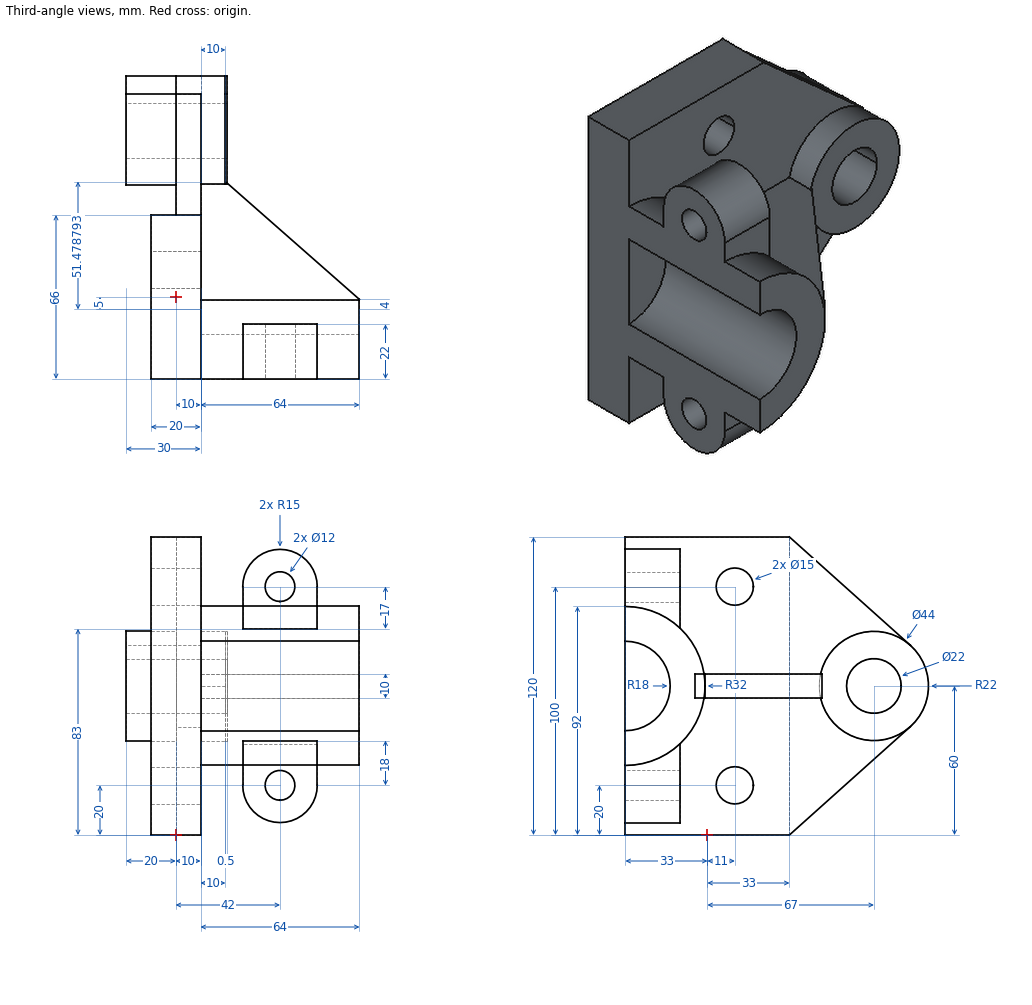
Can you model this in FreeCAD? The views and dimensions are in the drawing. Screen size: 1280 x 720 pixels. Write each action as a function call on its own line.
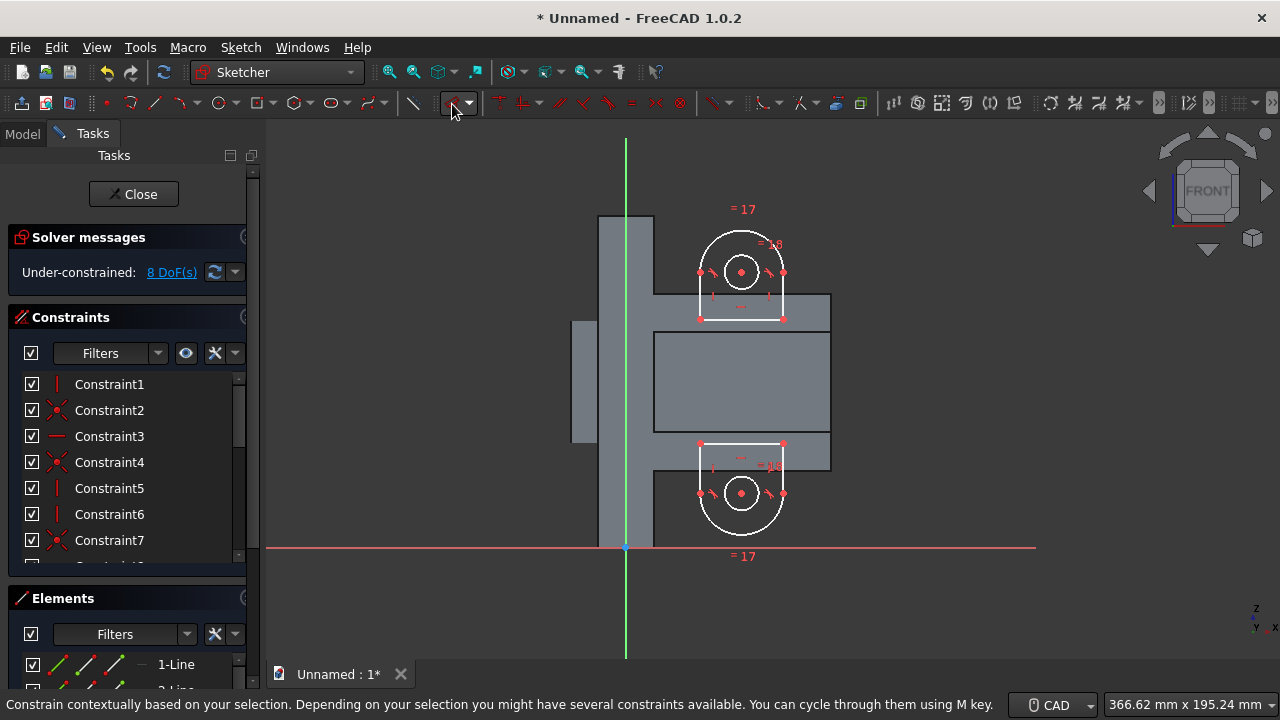
click(766, 239)
click(785, 213)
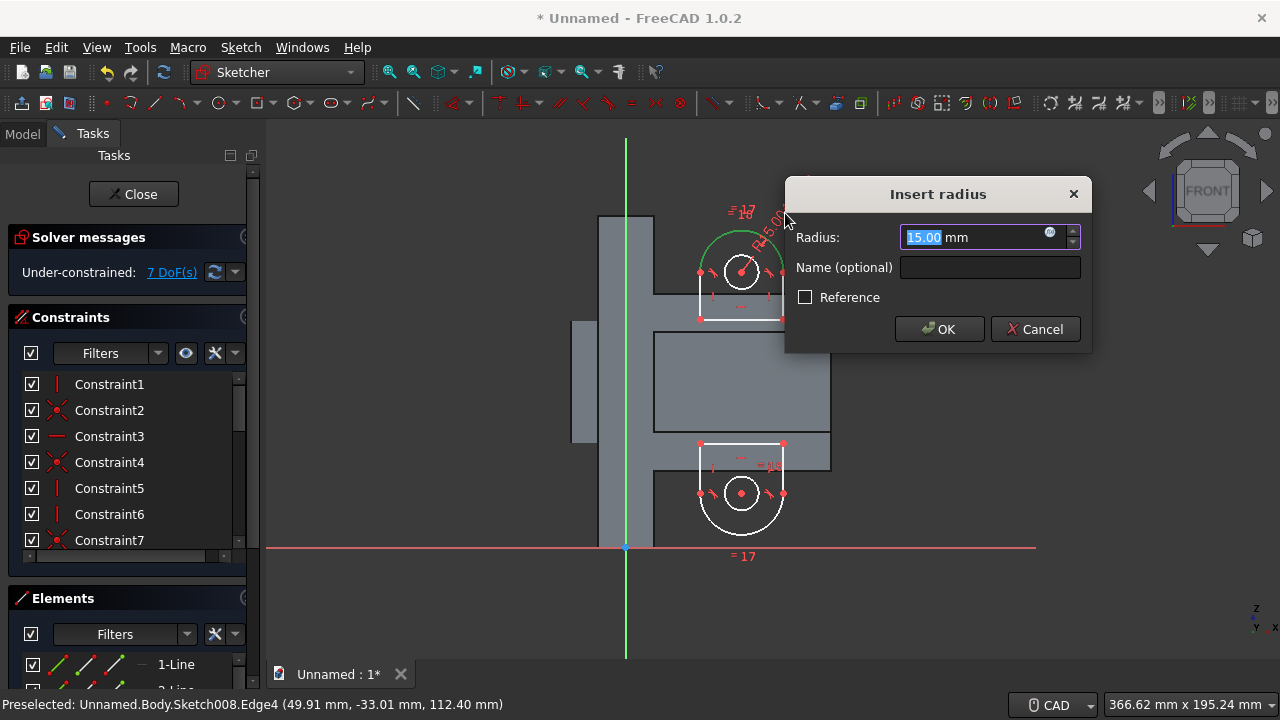
text(15)
key(Return)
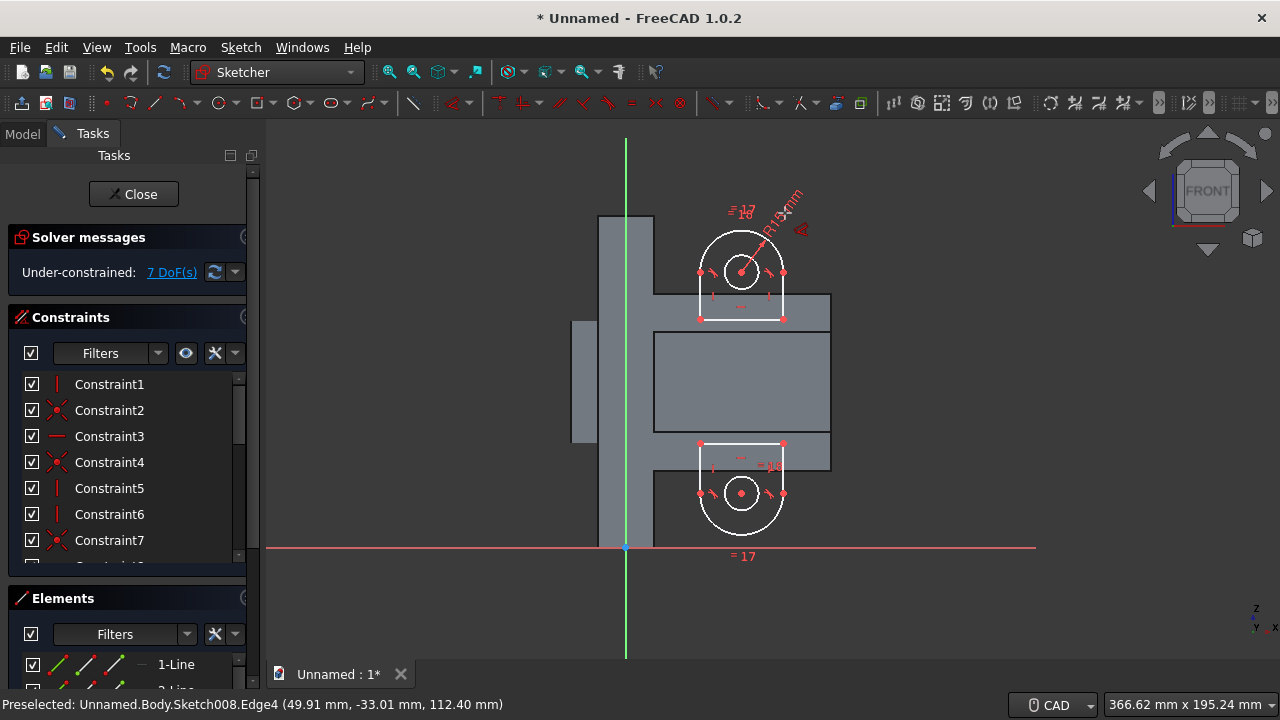
click(754, 260)
click(811, 252)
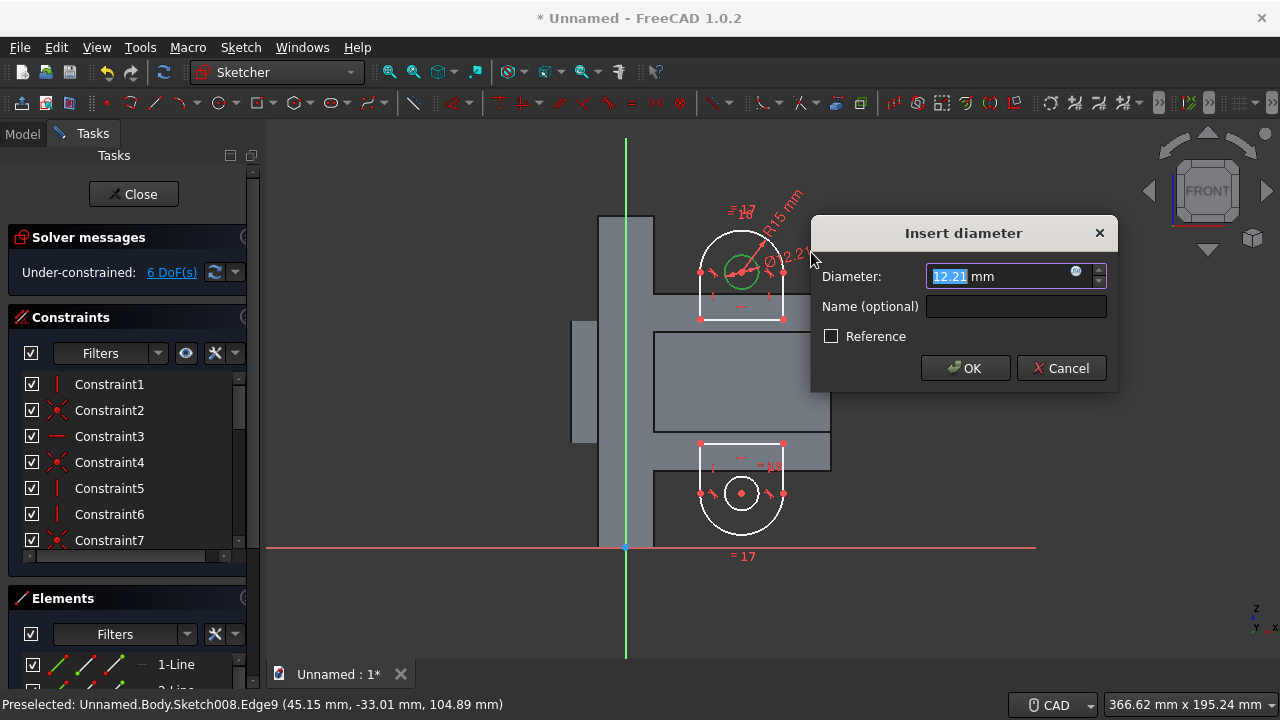
text(12)
key(Return)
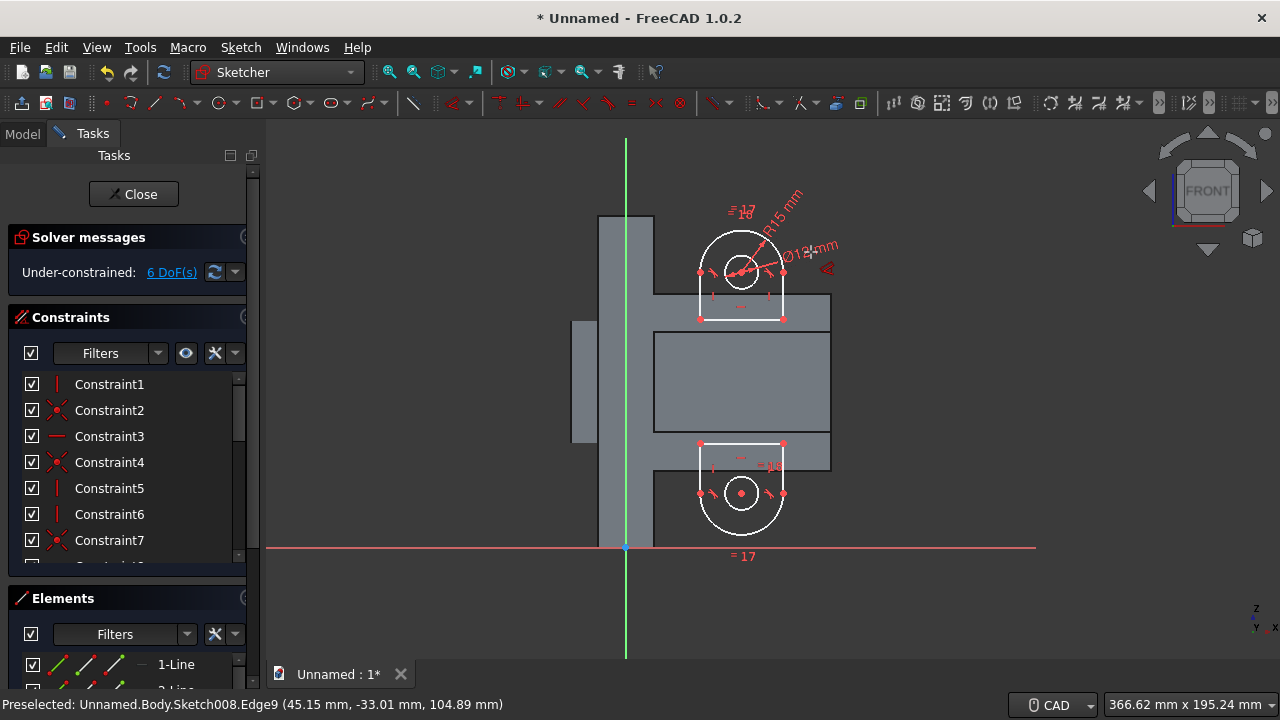
click(700, 286)
click(666, 296)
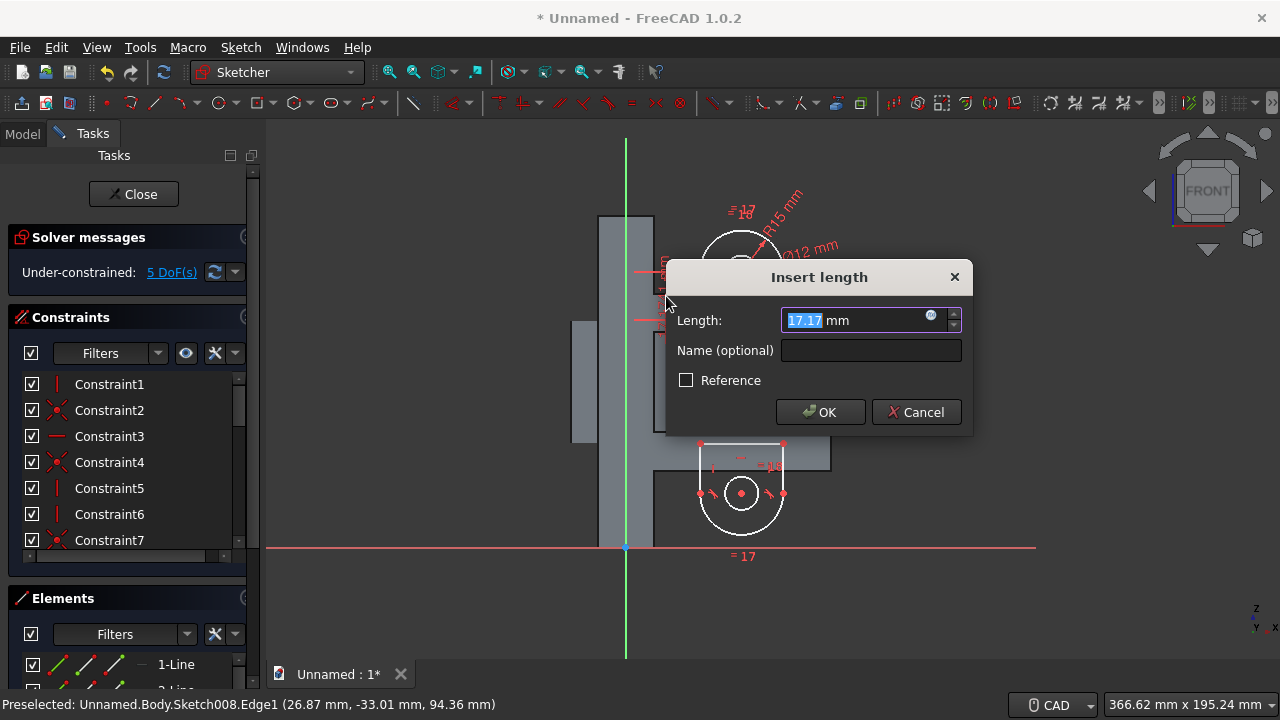
text(17)
key(Return)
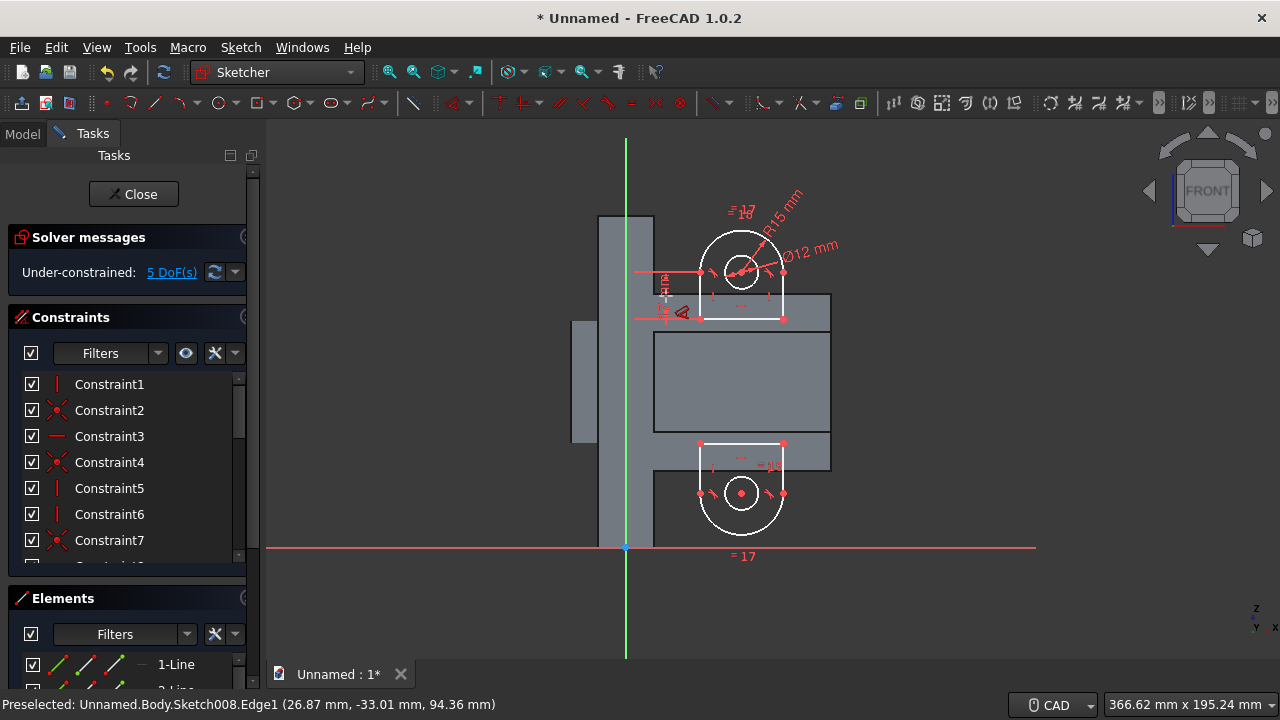
click(783, 478)
click(817, 469)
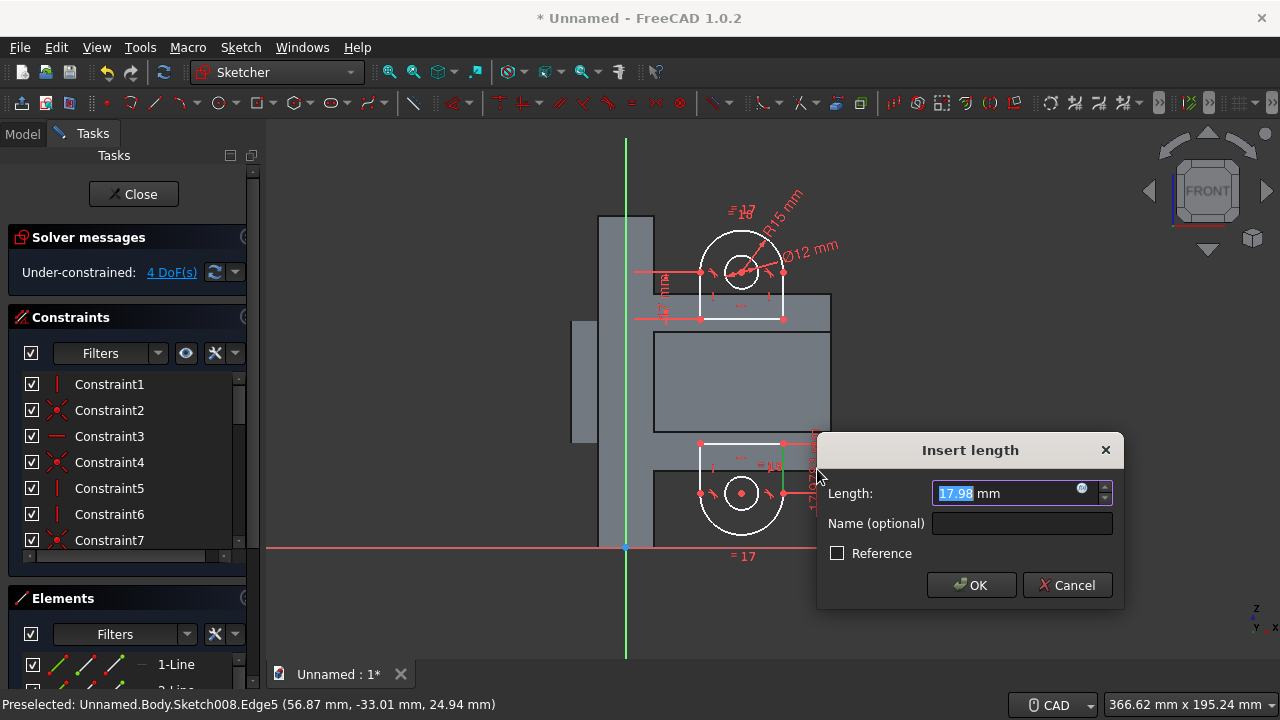
text(18)
key(Return)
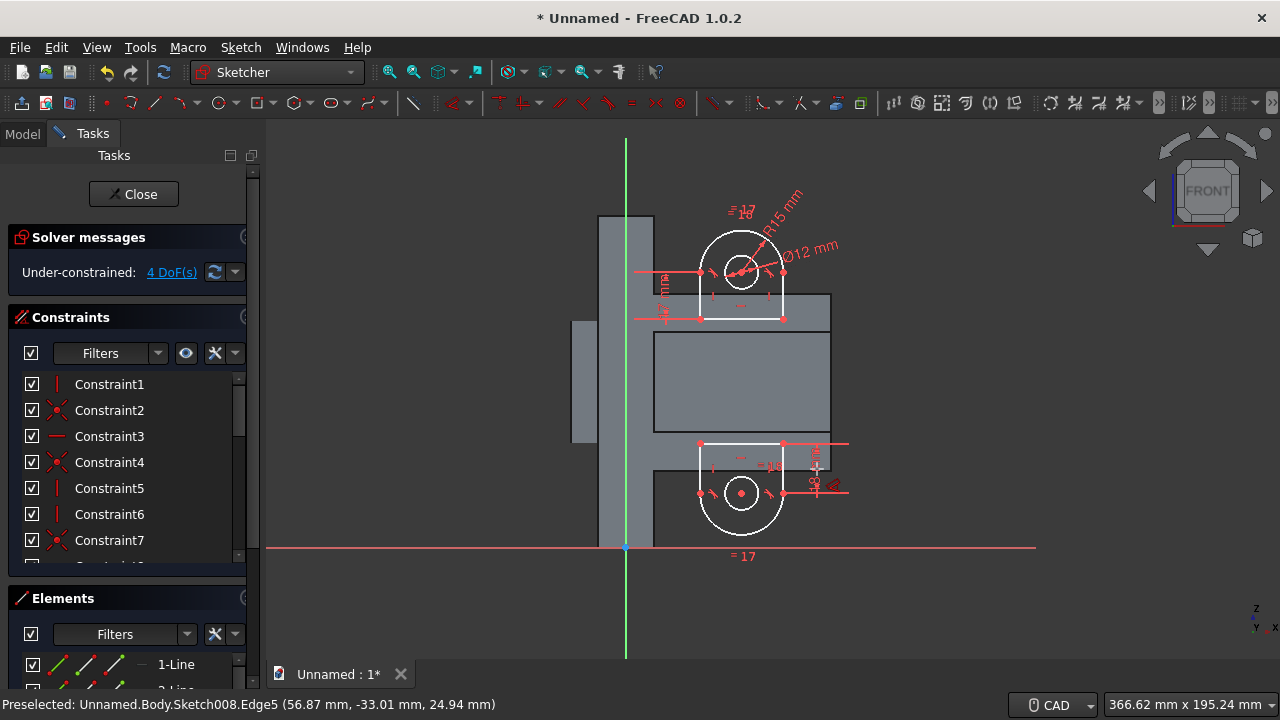
click(742, 272)
click(684, 582)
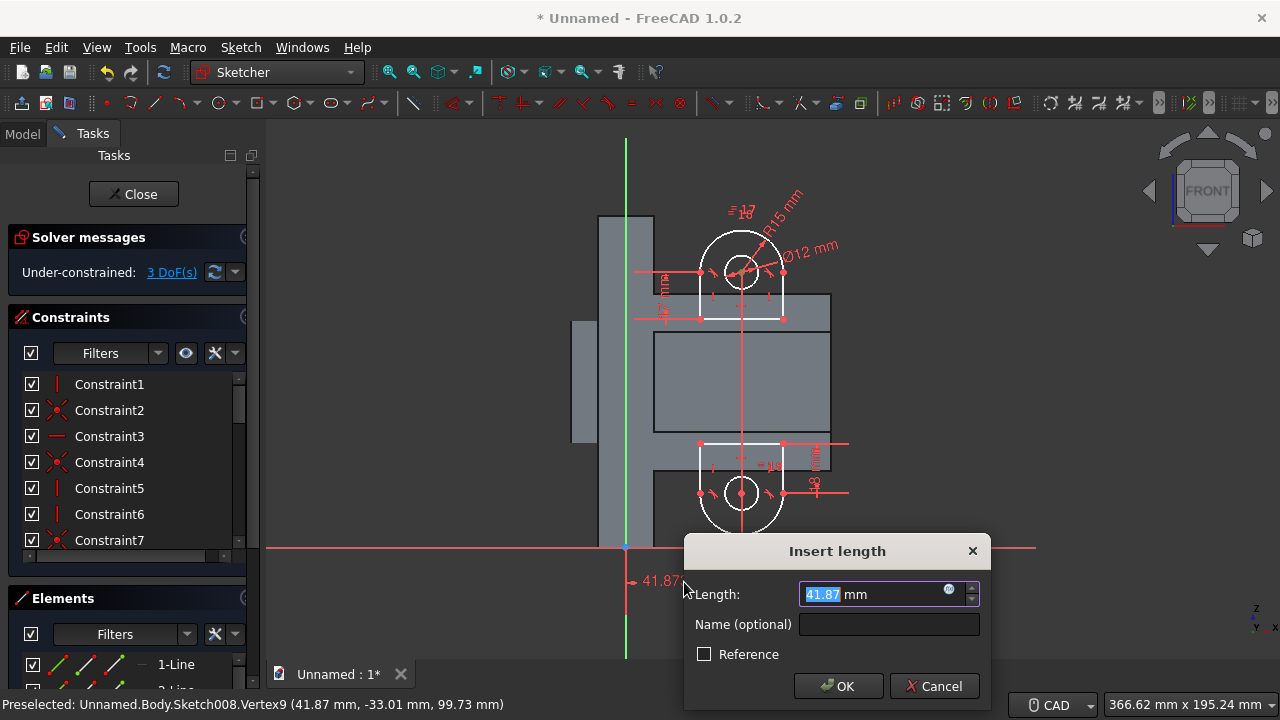
text(42)
key(Return)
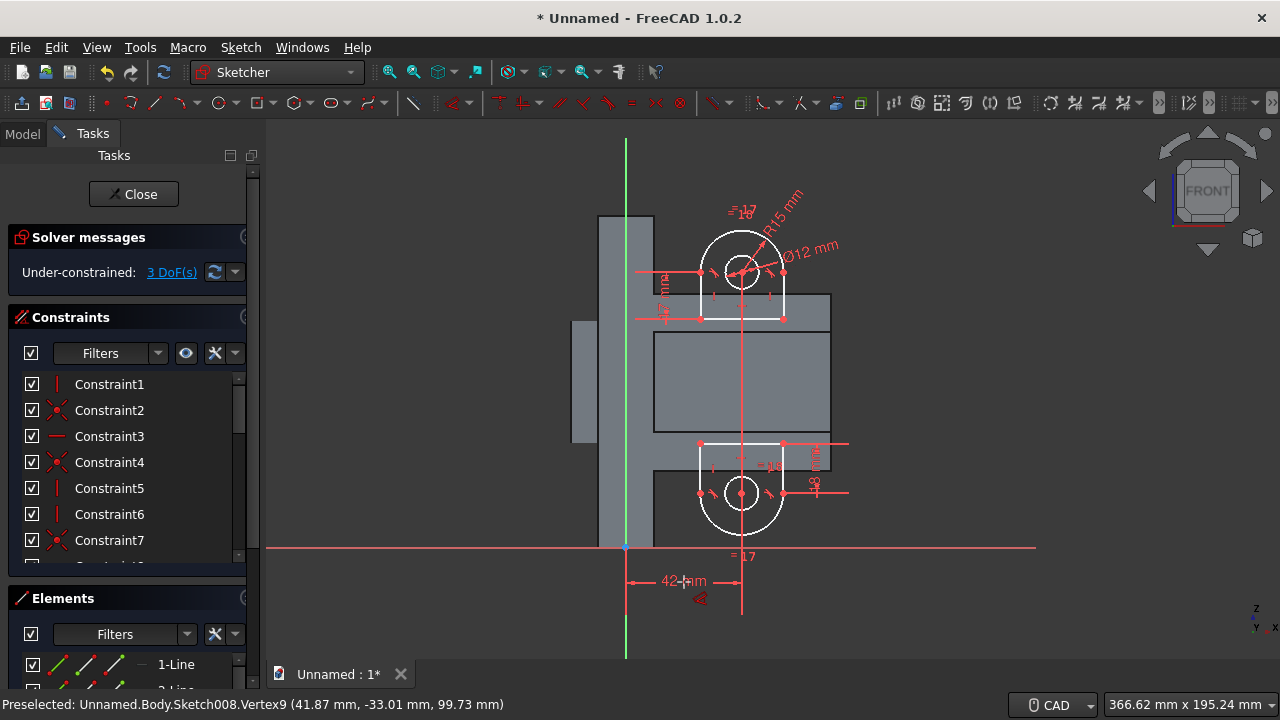
click(742, 493)
click(684, 459)